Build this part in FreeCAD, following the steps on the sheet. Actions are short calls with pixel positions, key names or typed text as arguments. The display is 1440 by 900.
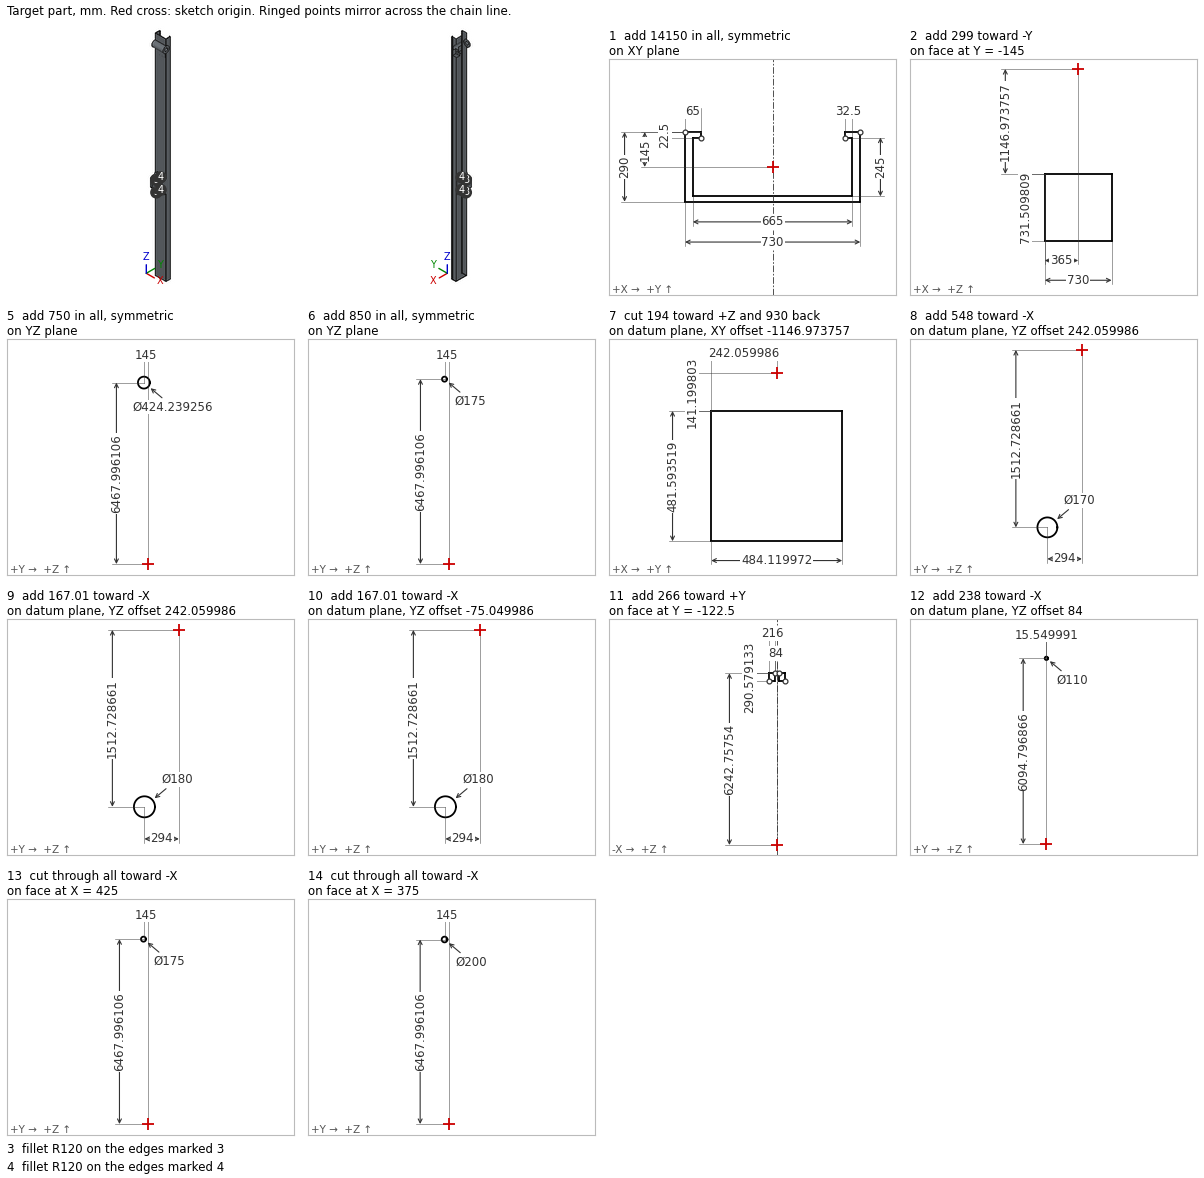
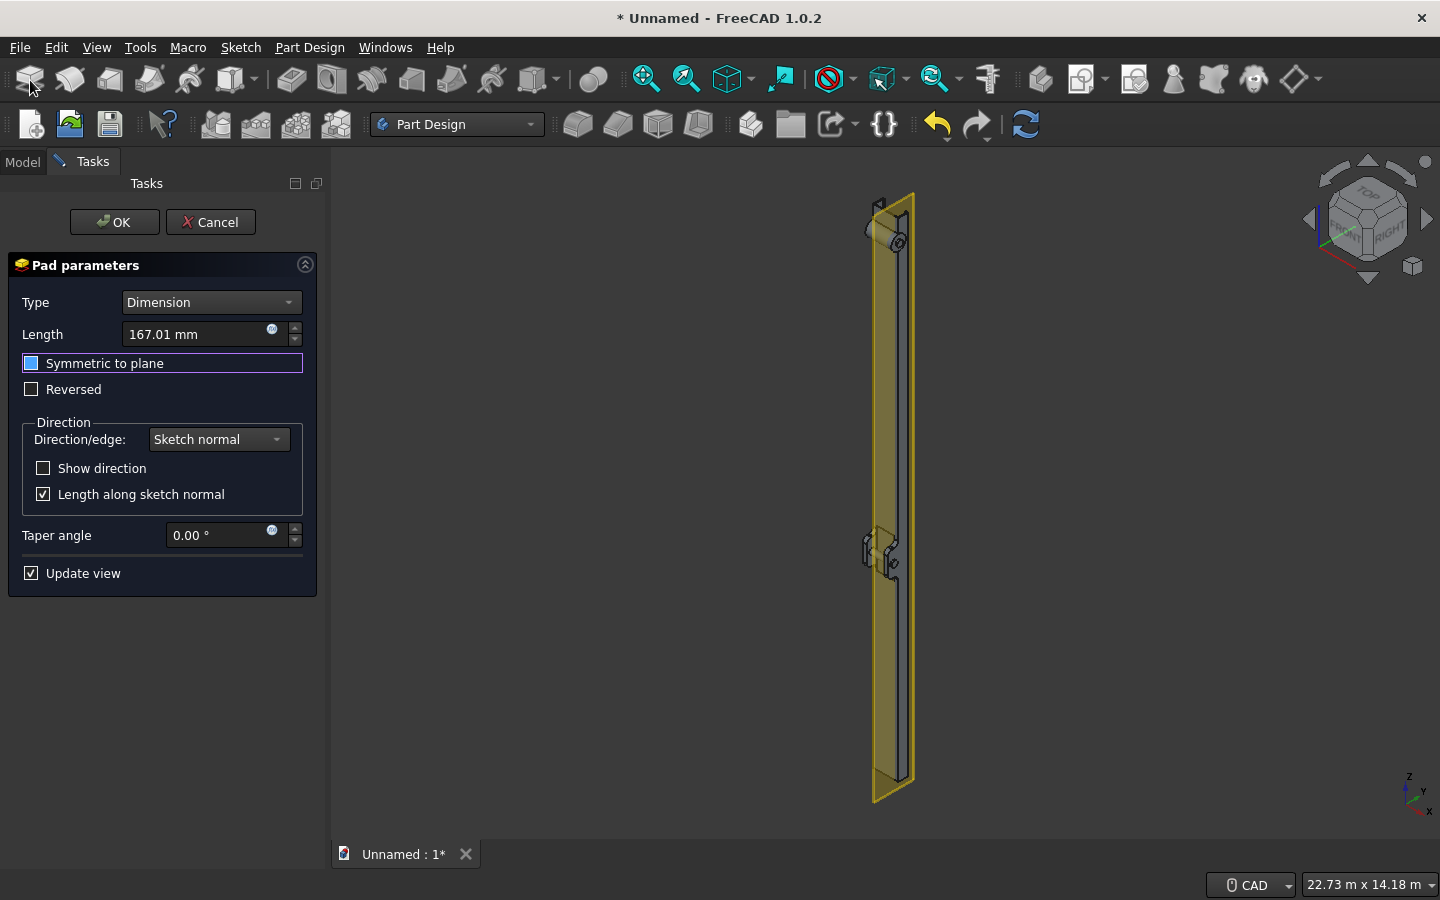
click(30, 389)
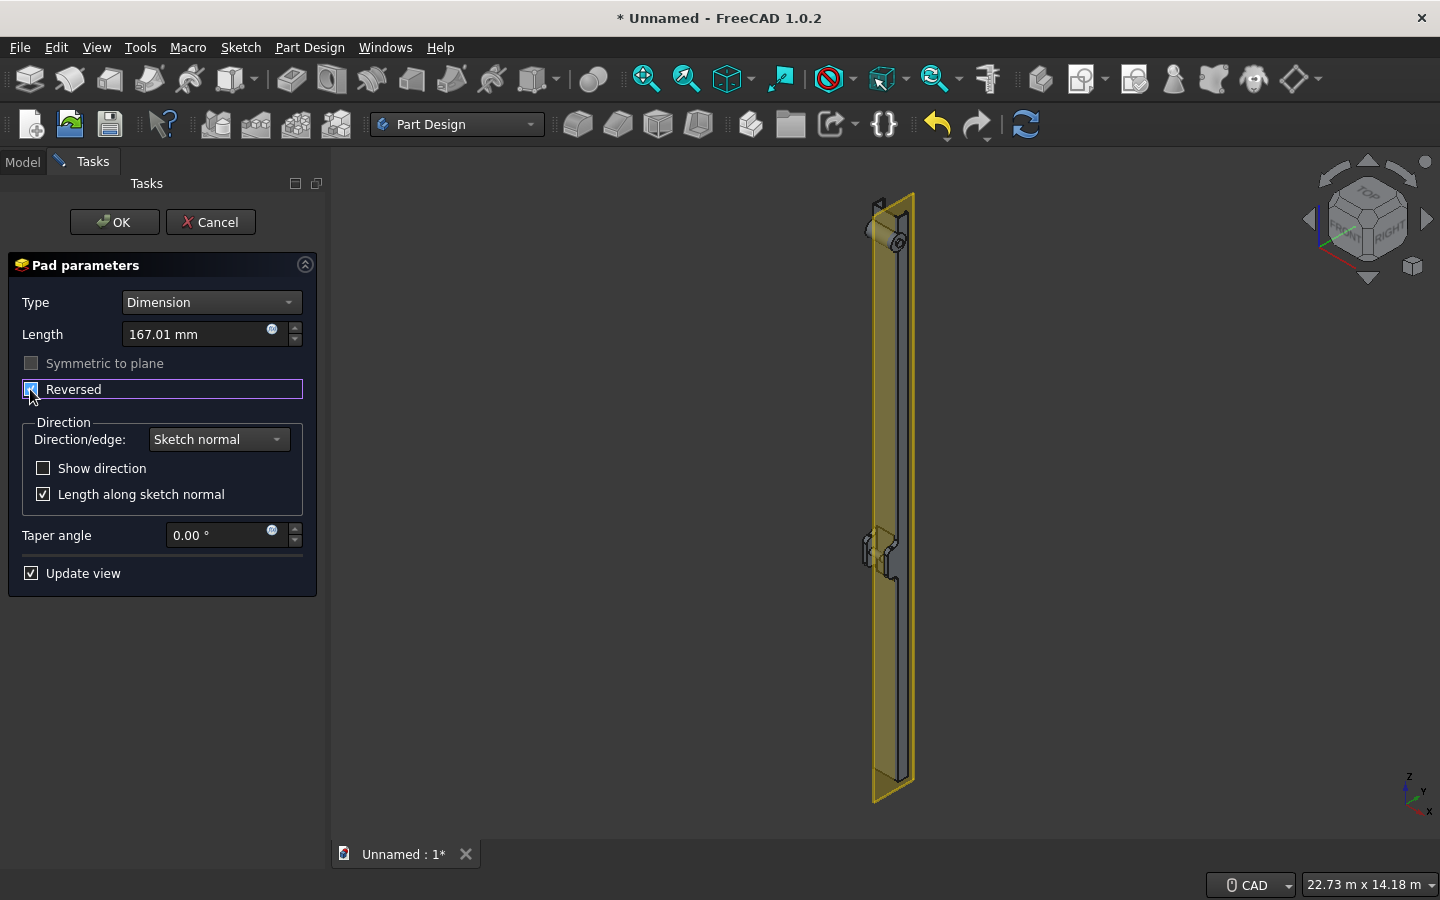
click(115, 222)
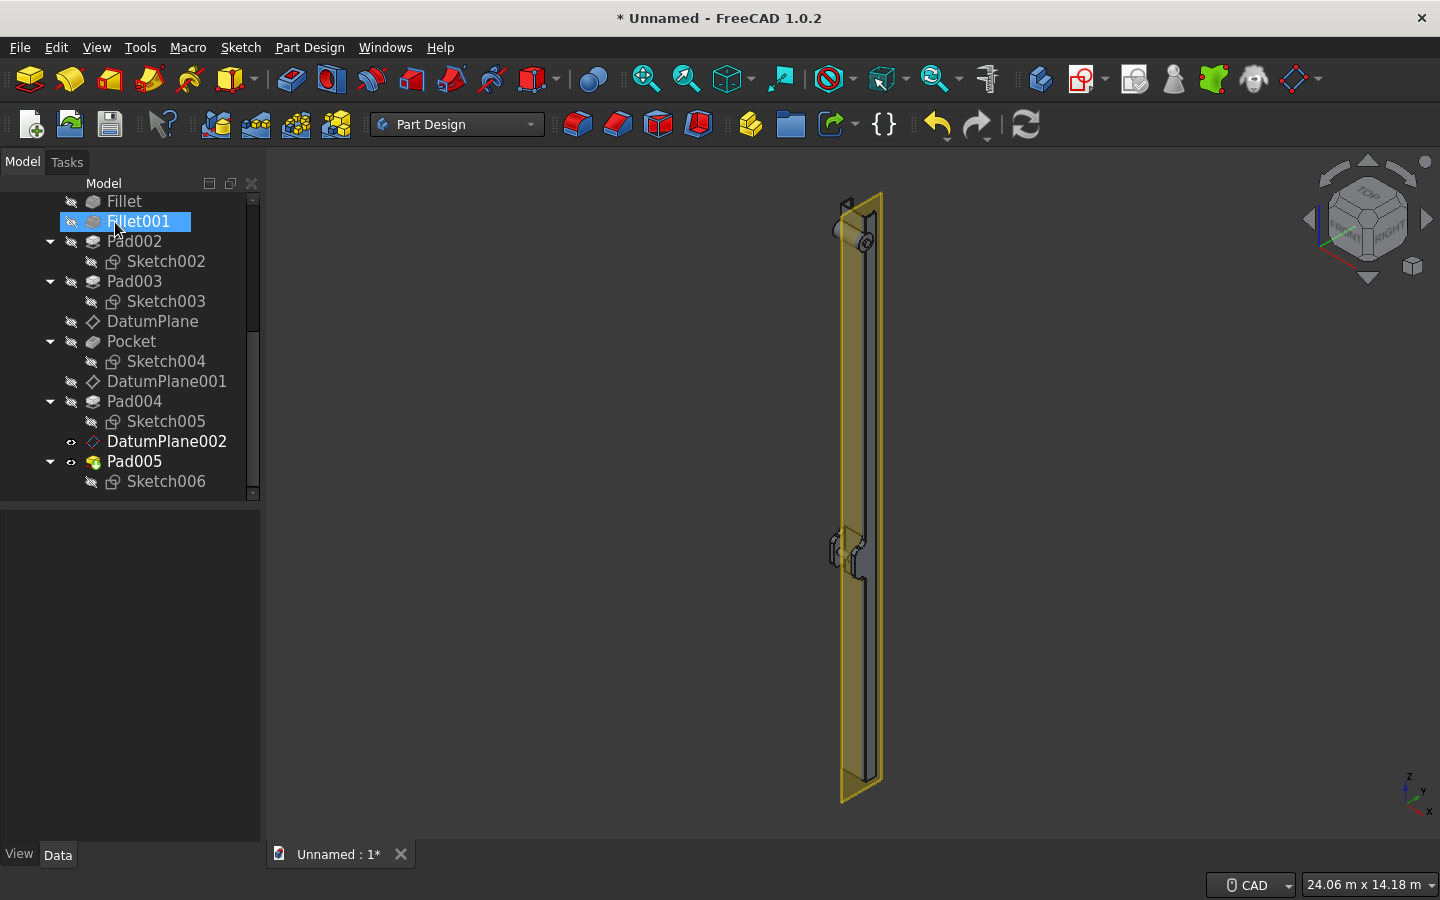
click(116, 442)
key(space)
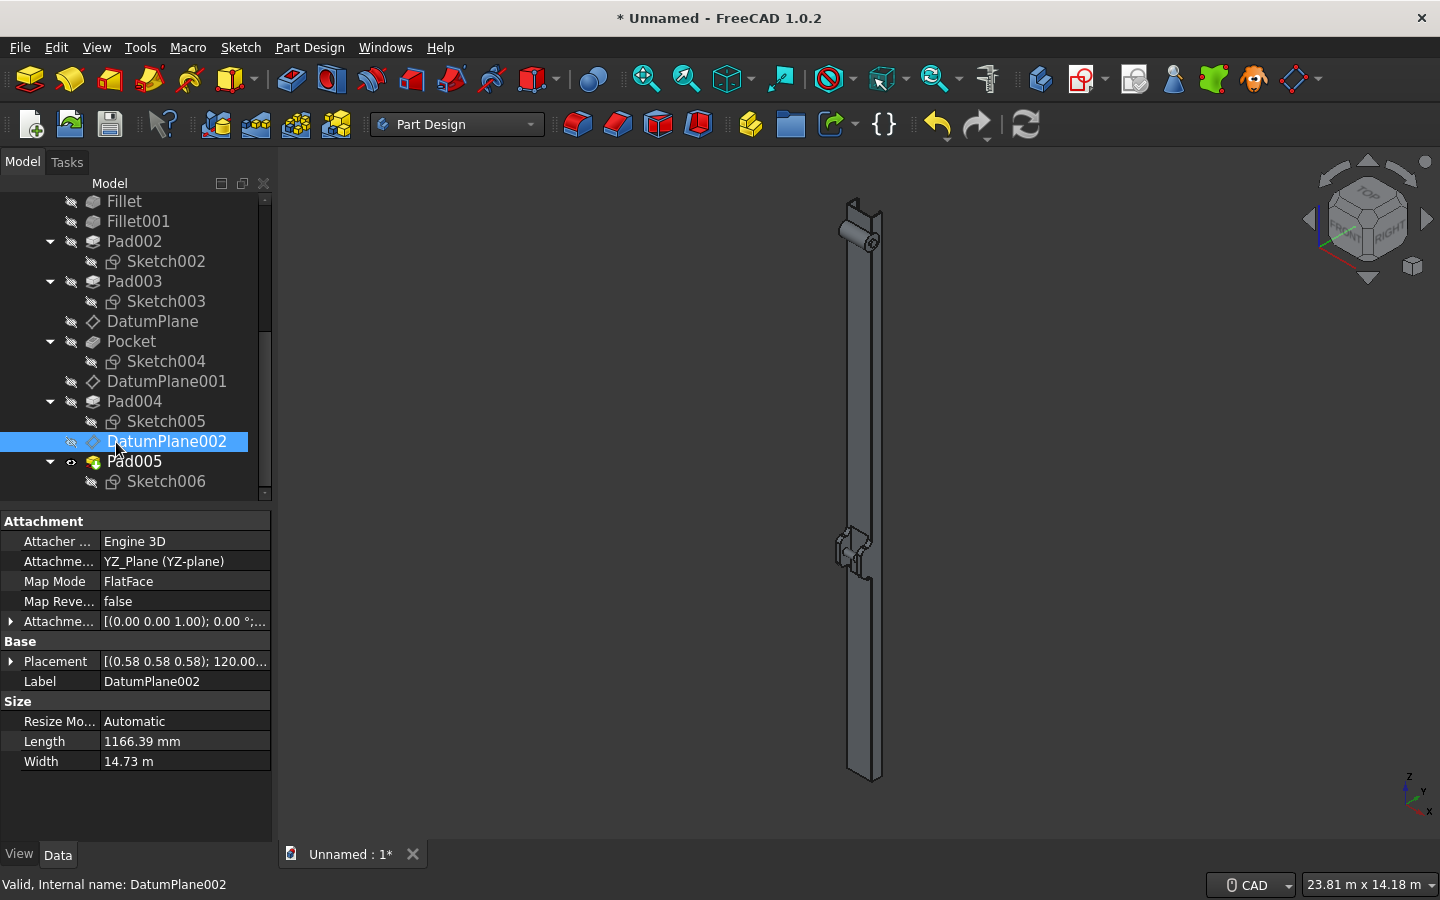
scroll(140, 337, down, 3)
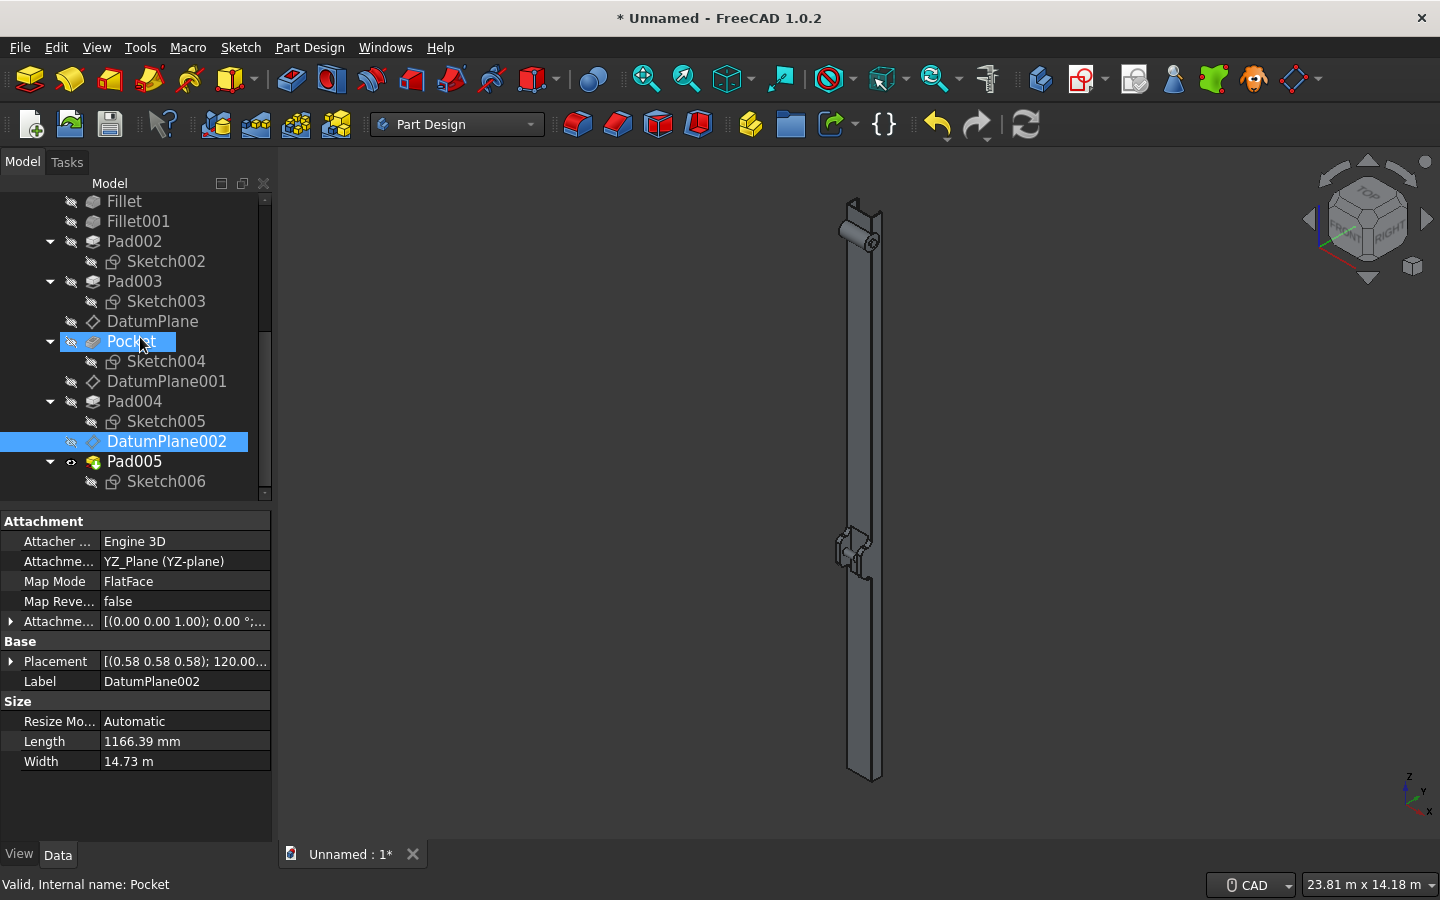
scroll(140, 337, up, 15)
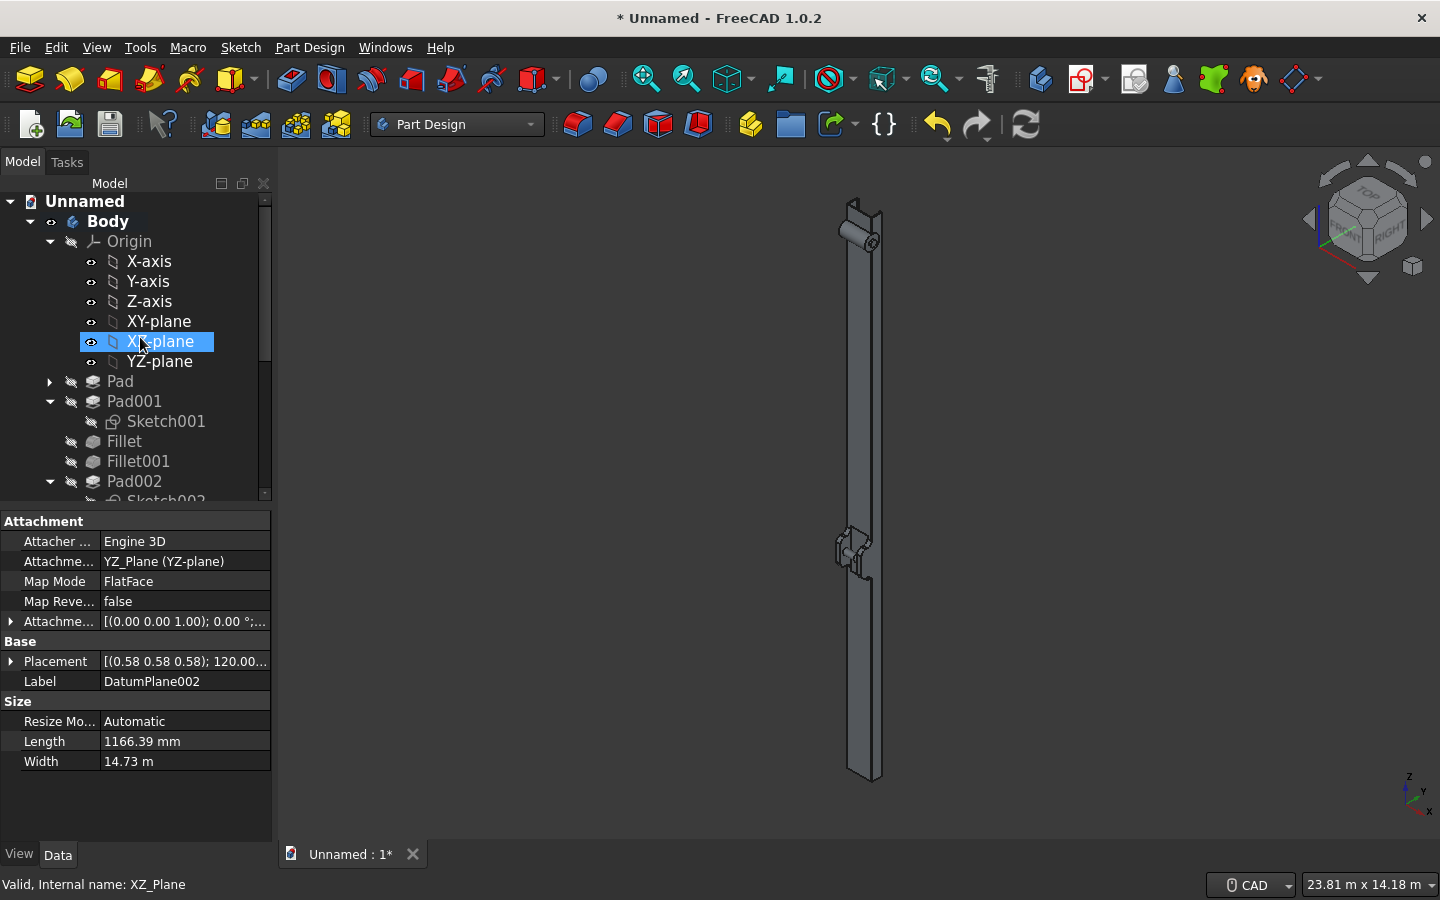
click(136, 362)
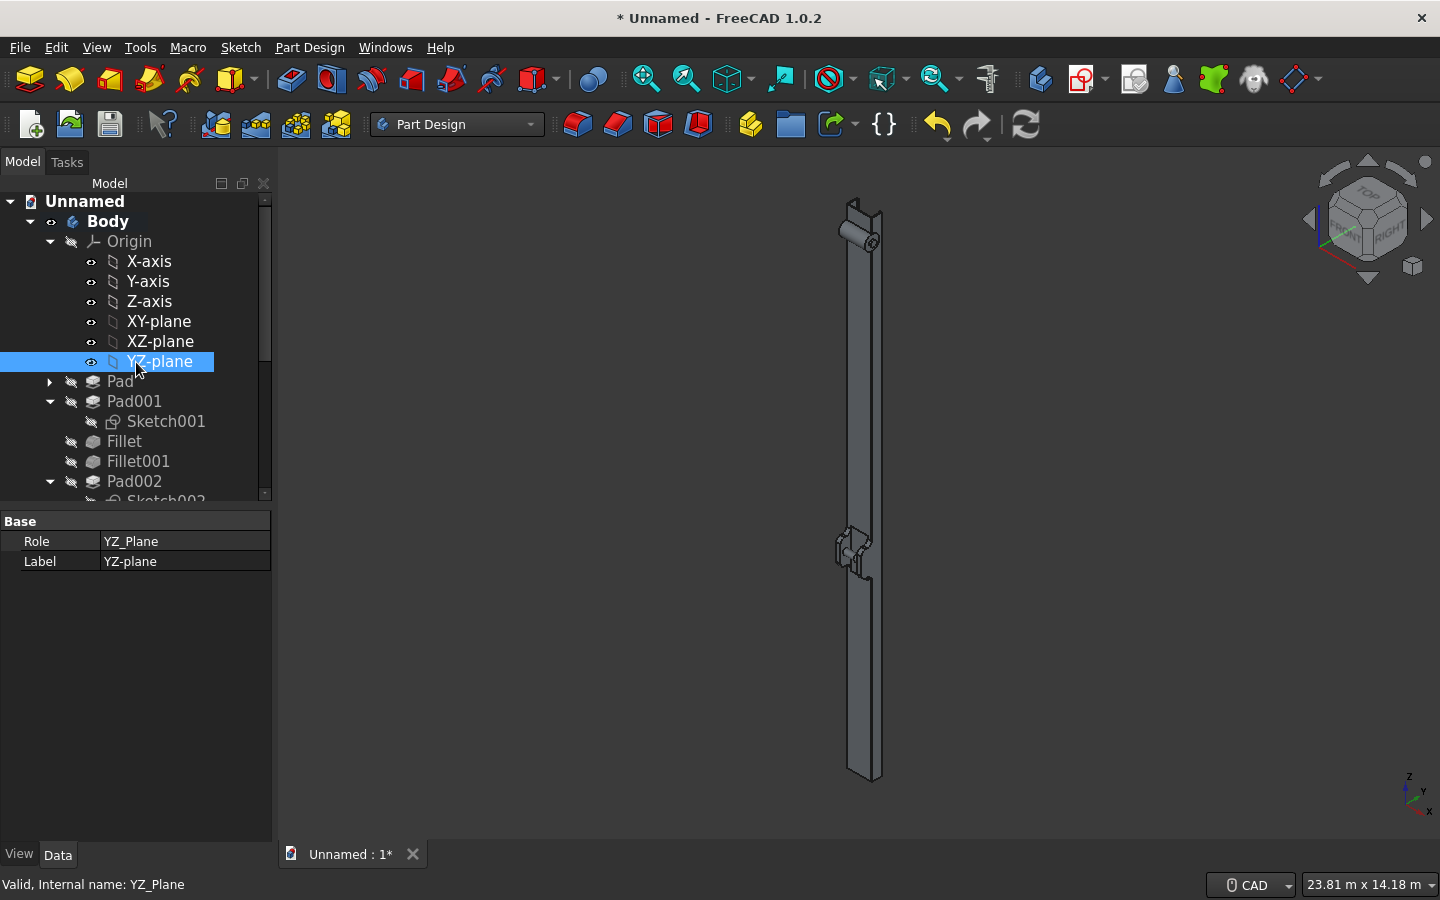
click(1294, 80)